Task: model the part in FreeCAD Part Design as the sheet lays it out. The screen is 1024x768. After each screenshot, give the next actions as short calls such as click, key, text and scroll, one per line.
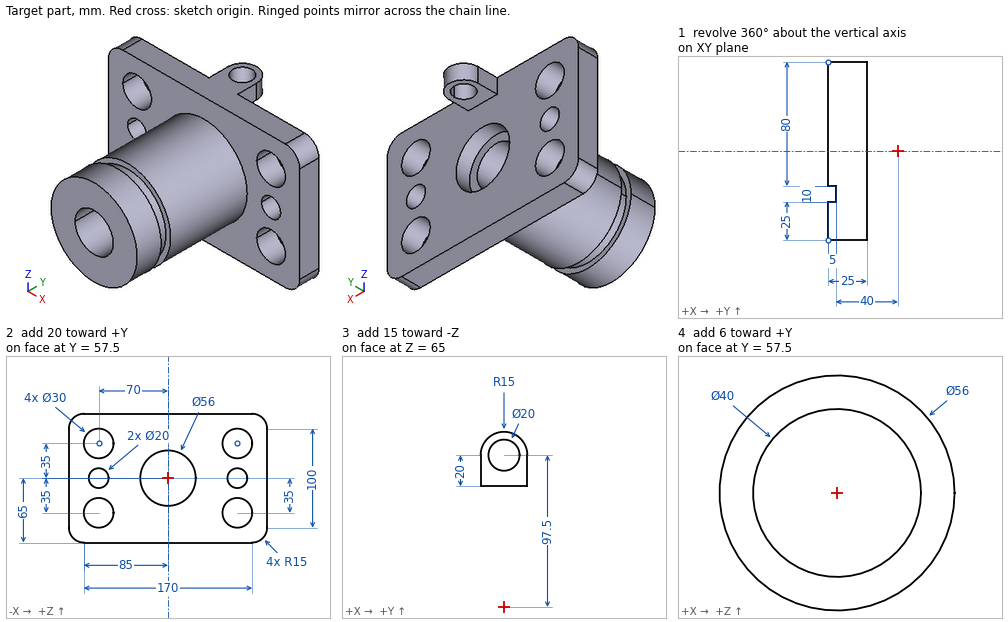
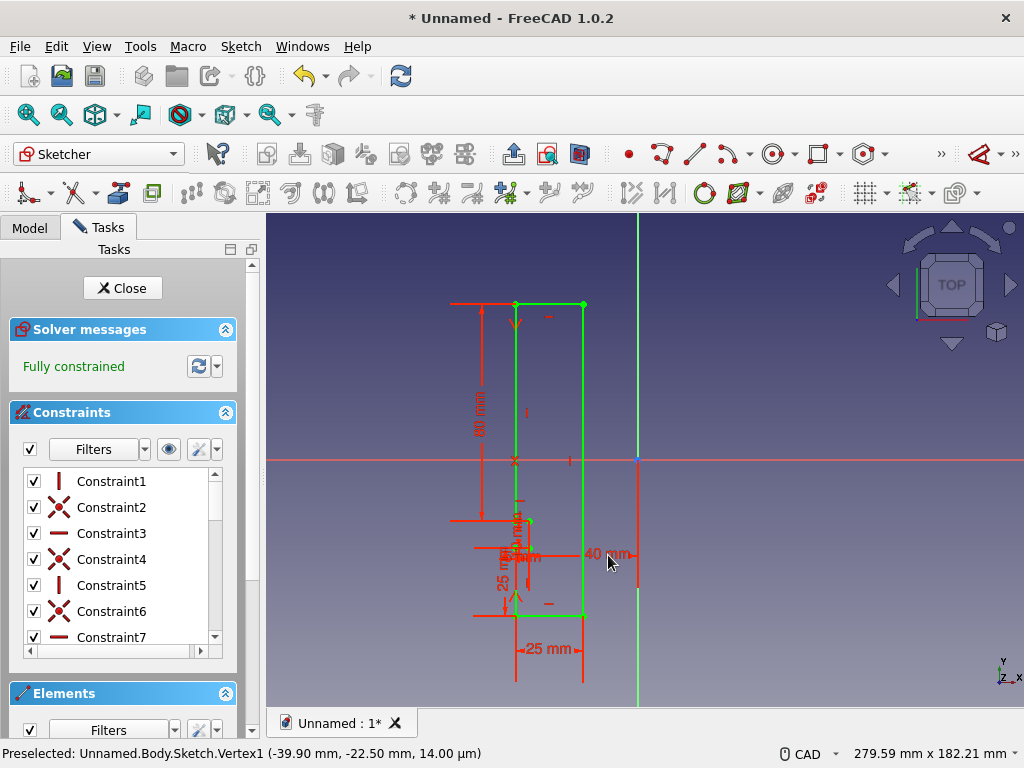
click(123, 288)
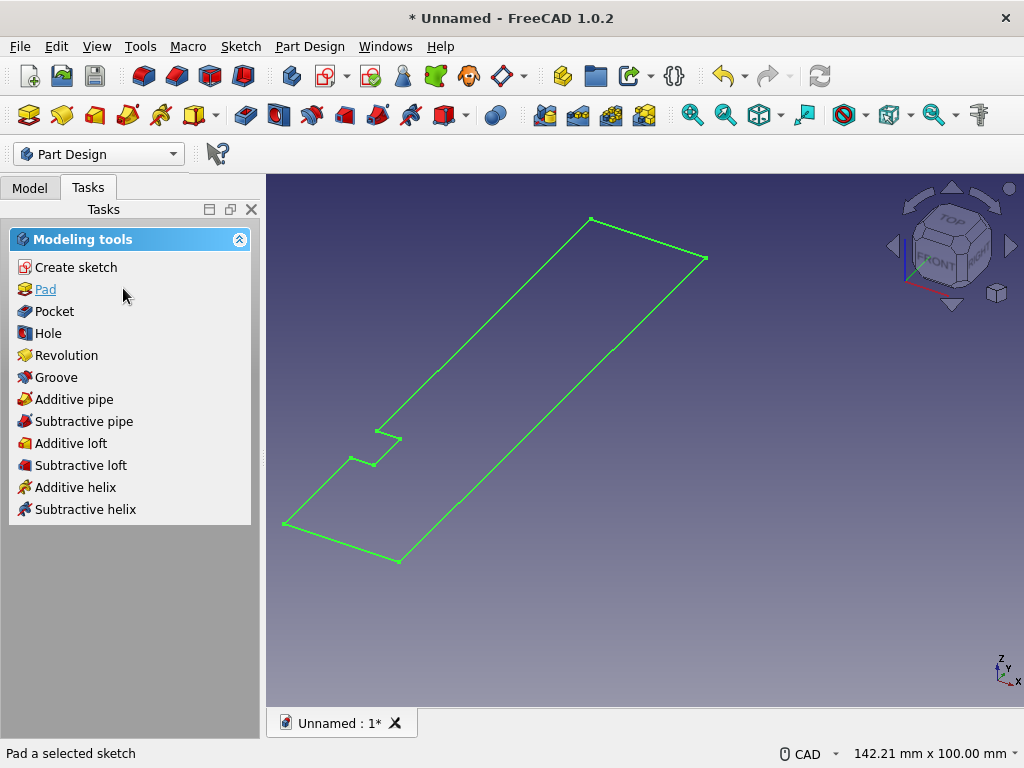
click(62, 116)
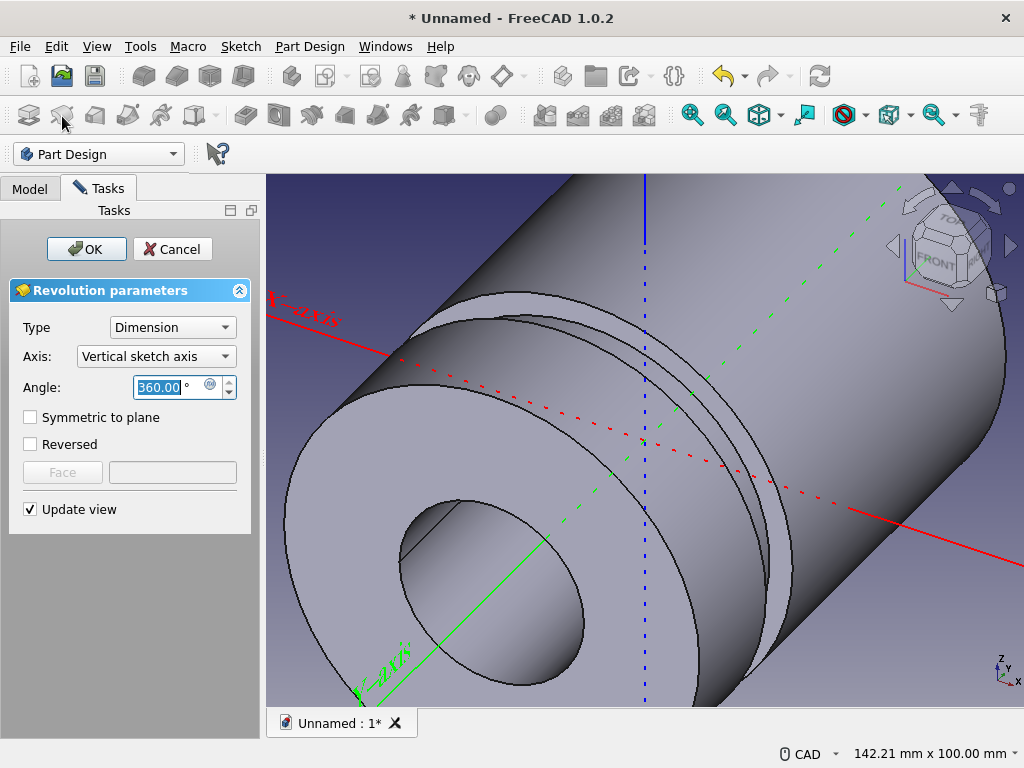
click(87, 249)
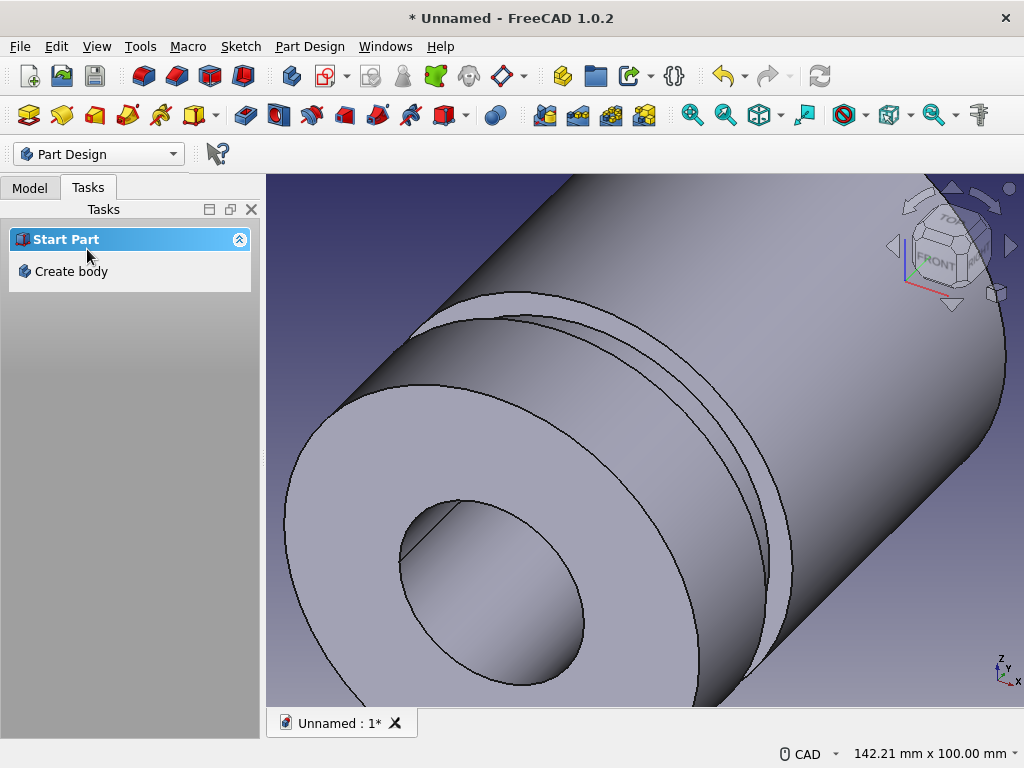
click(693, 116)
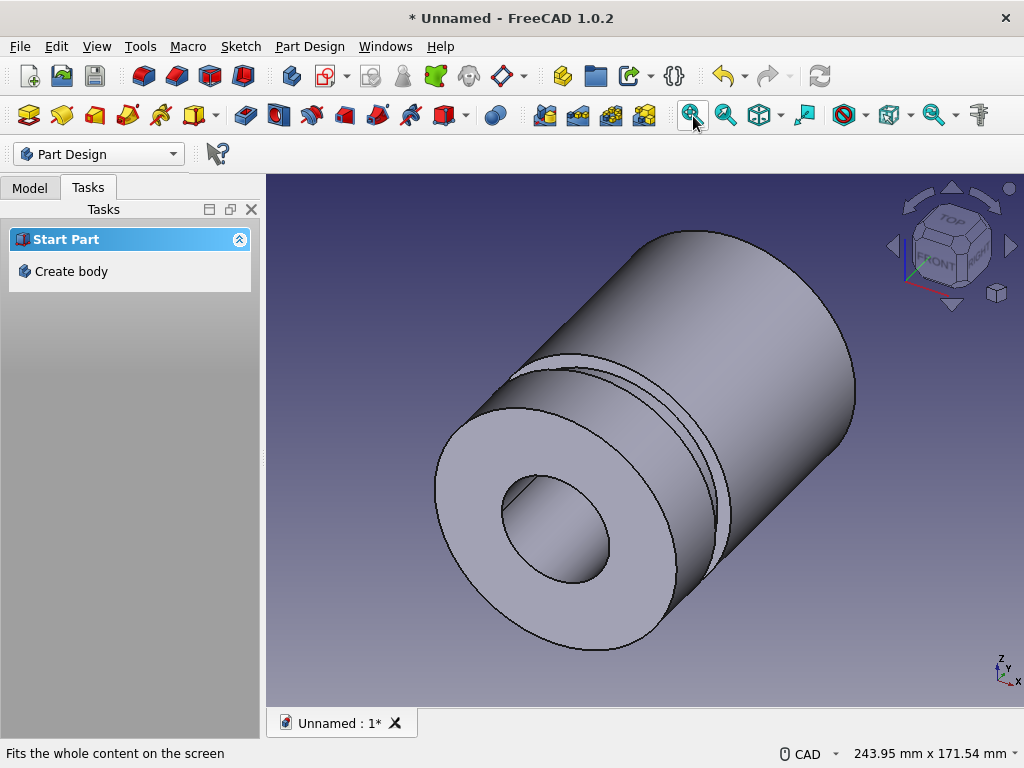
key(4)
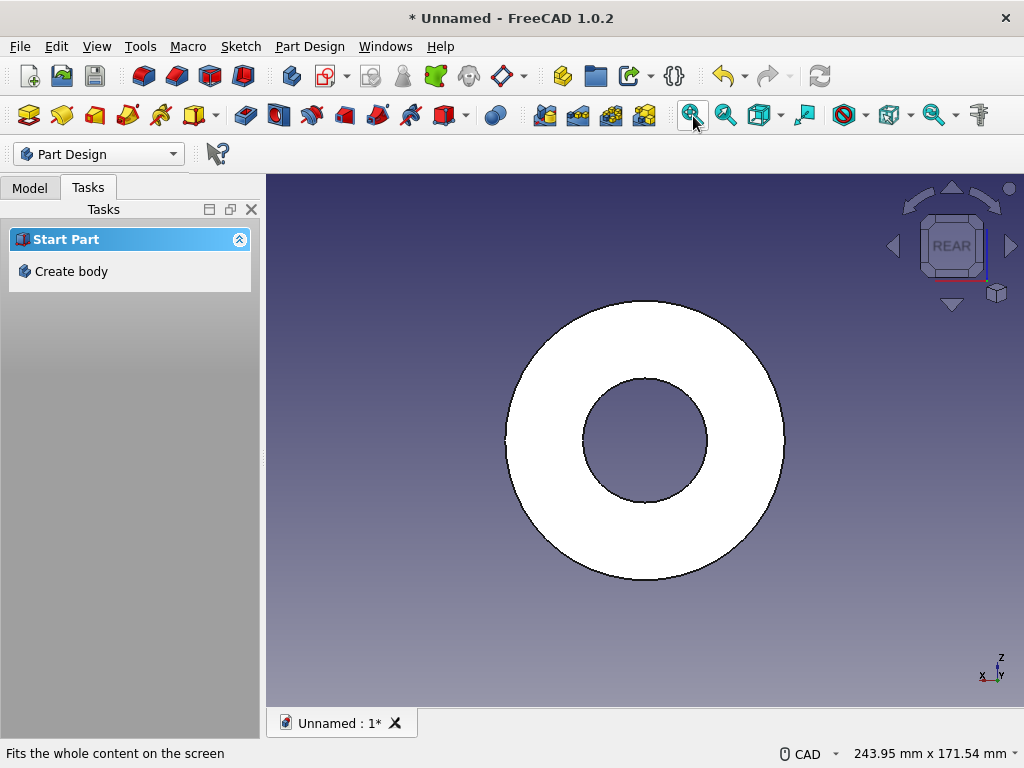
click(605, 519)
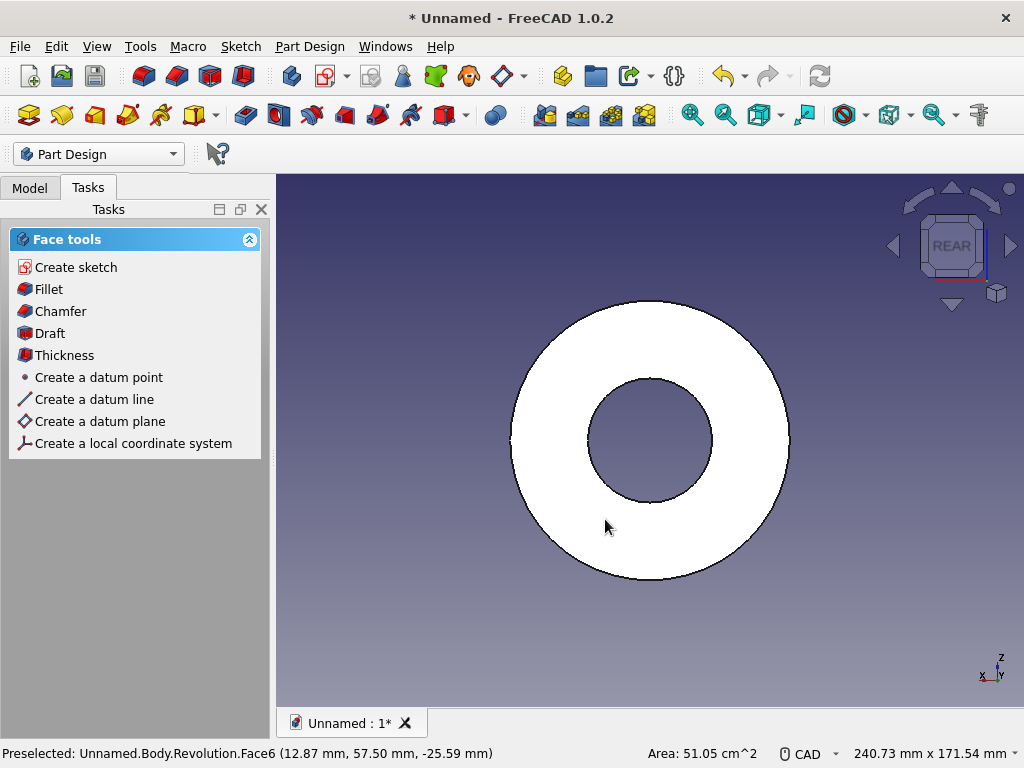
click(324, 76)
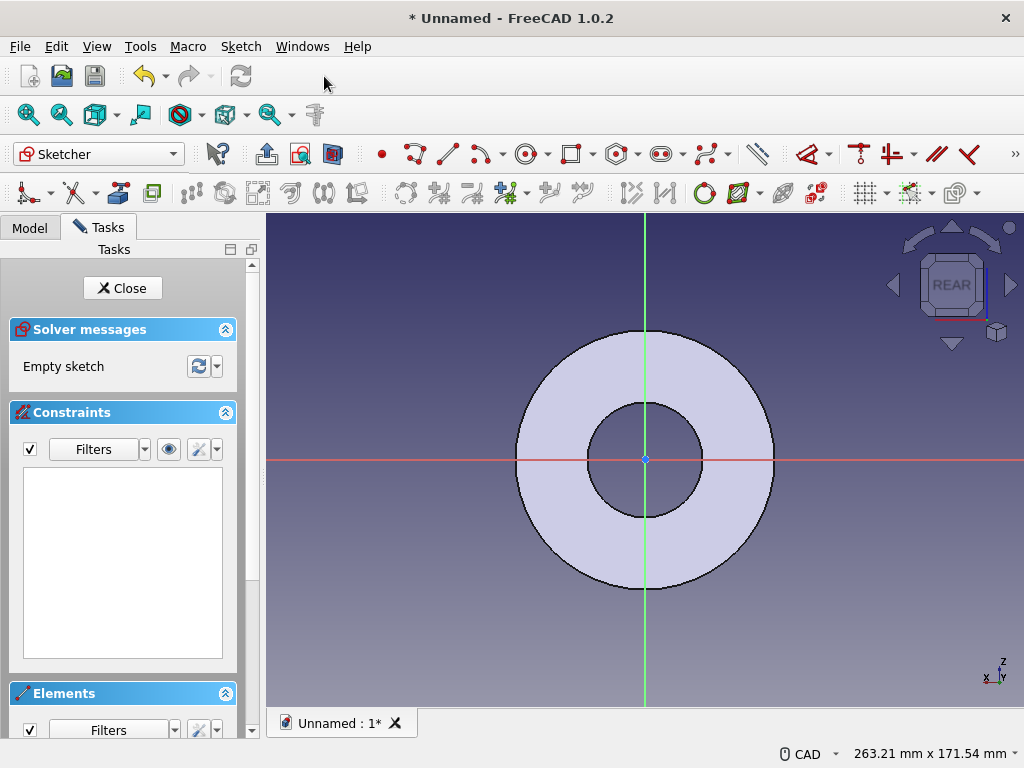
scroll(437, 460, down, 2)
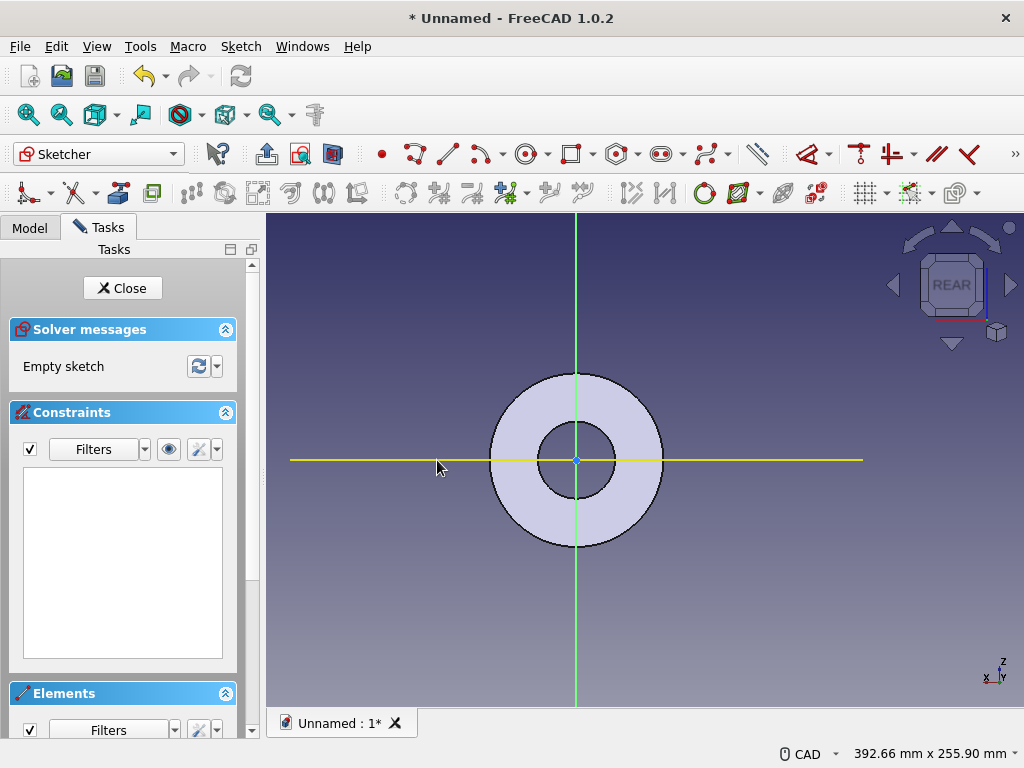
click(448, 154)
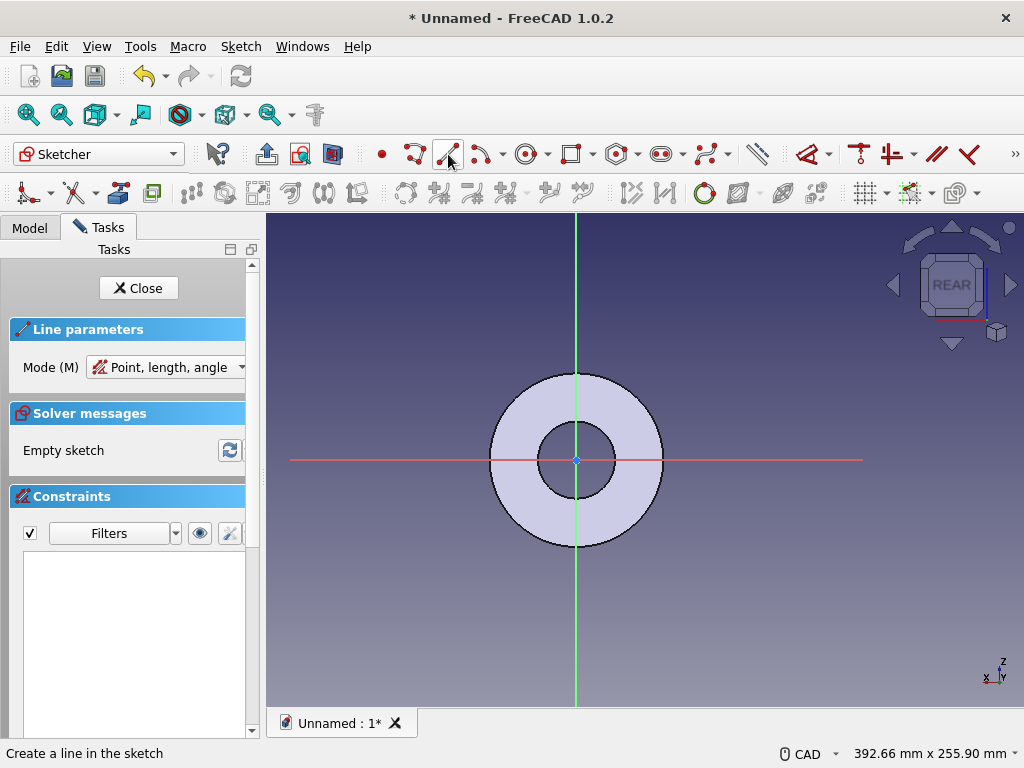
click(412, 586)
click(741, 586)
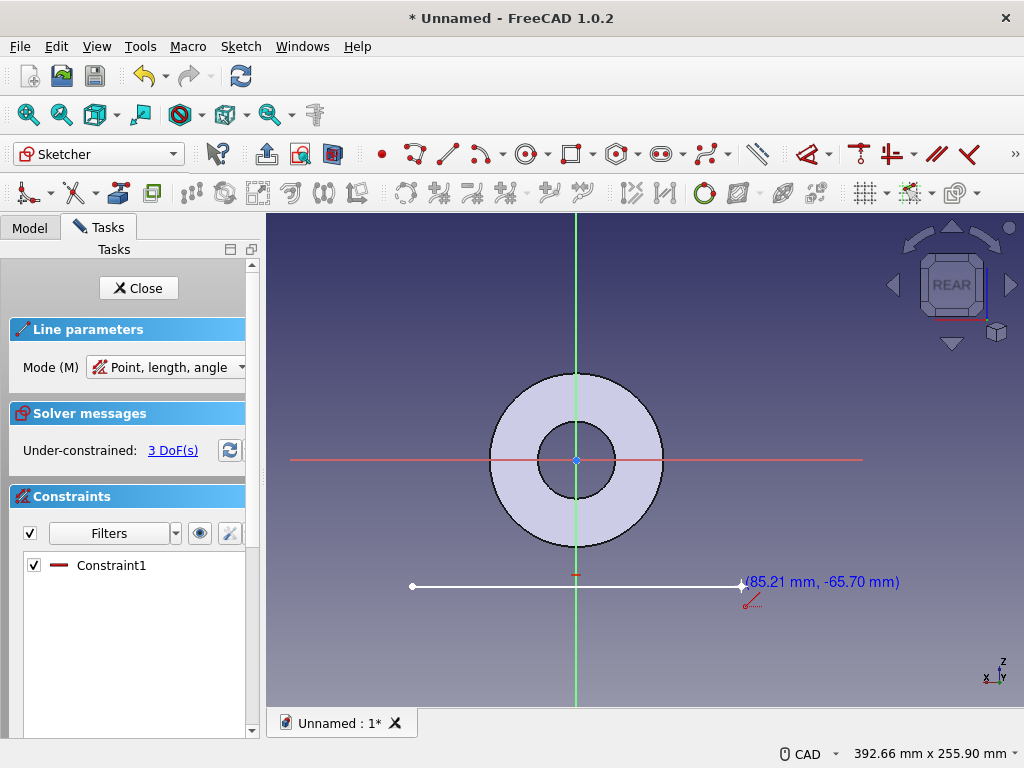
click(770, 557)
click(770, 364)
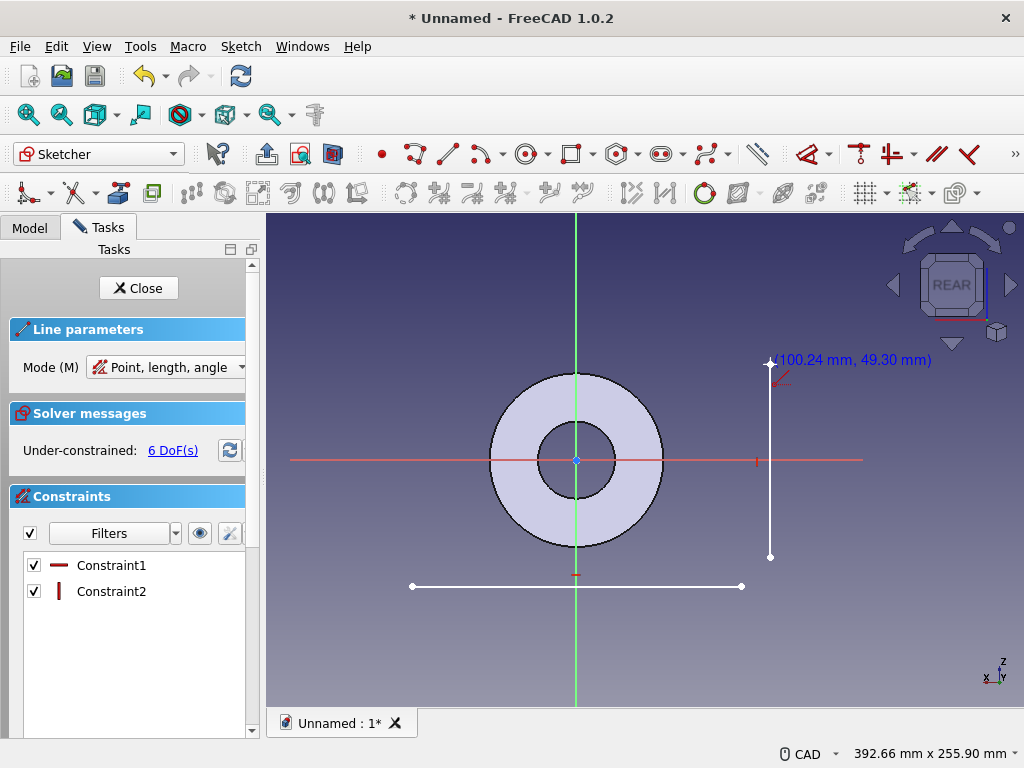
click(741, 335)
click(412, 335)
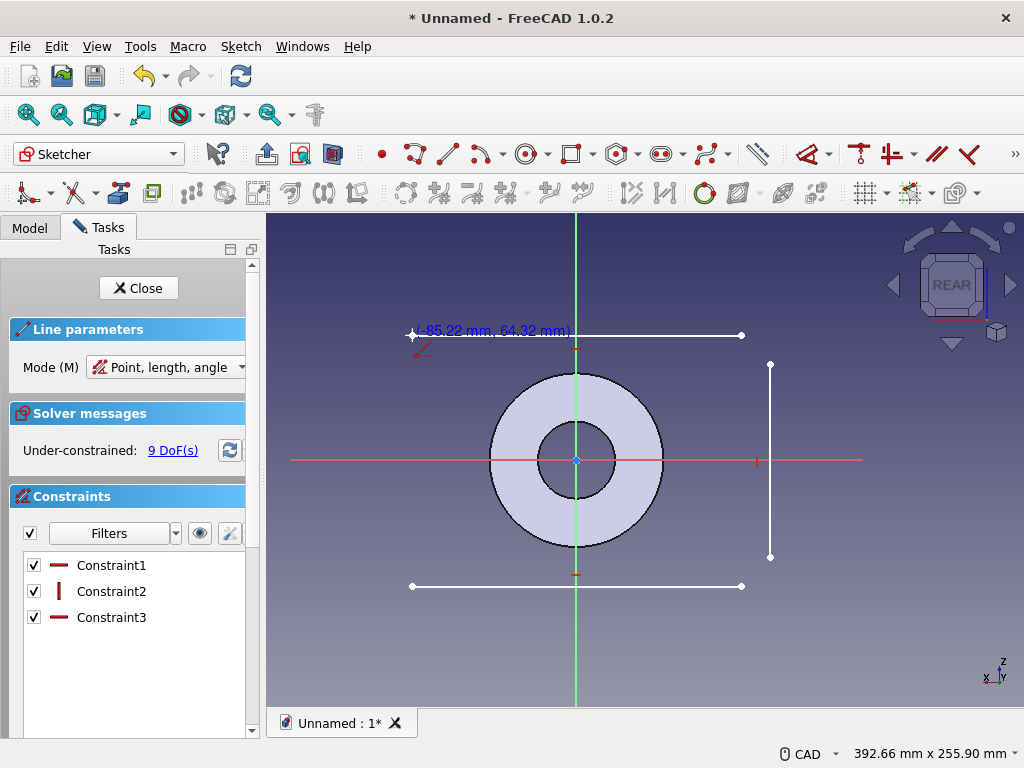
click(383, 364)
click(383, 557)